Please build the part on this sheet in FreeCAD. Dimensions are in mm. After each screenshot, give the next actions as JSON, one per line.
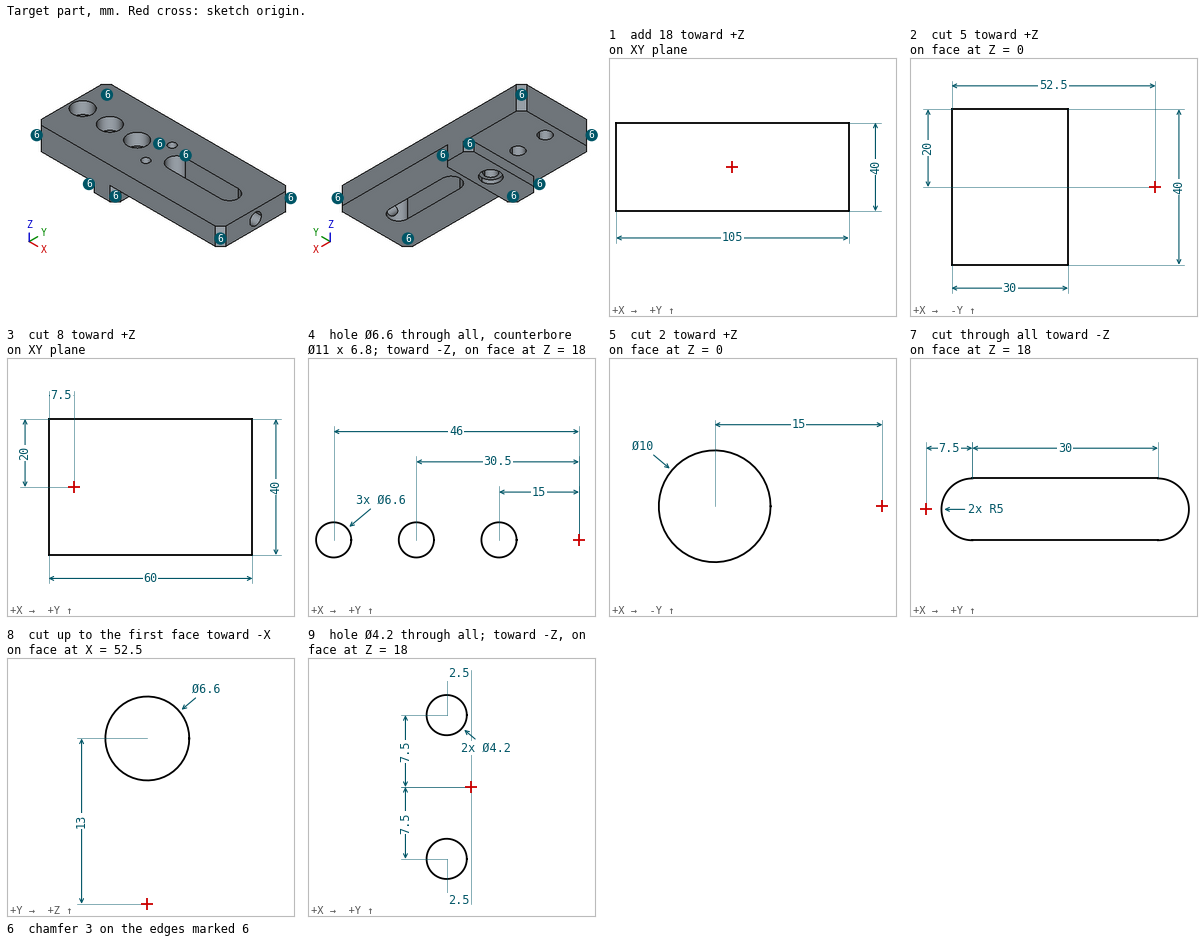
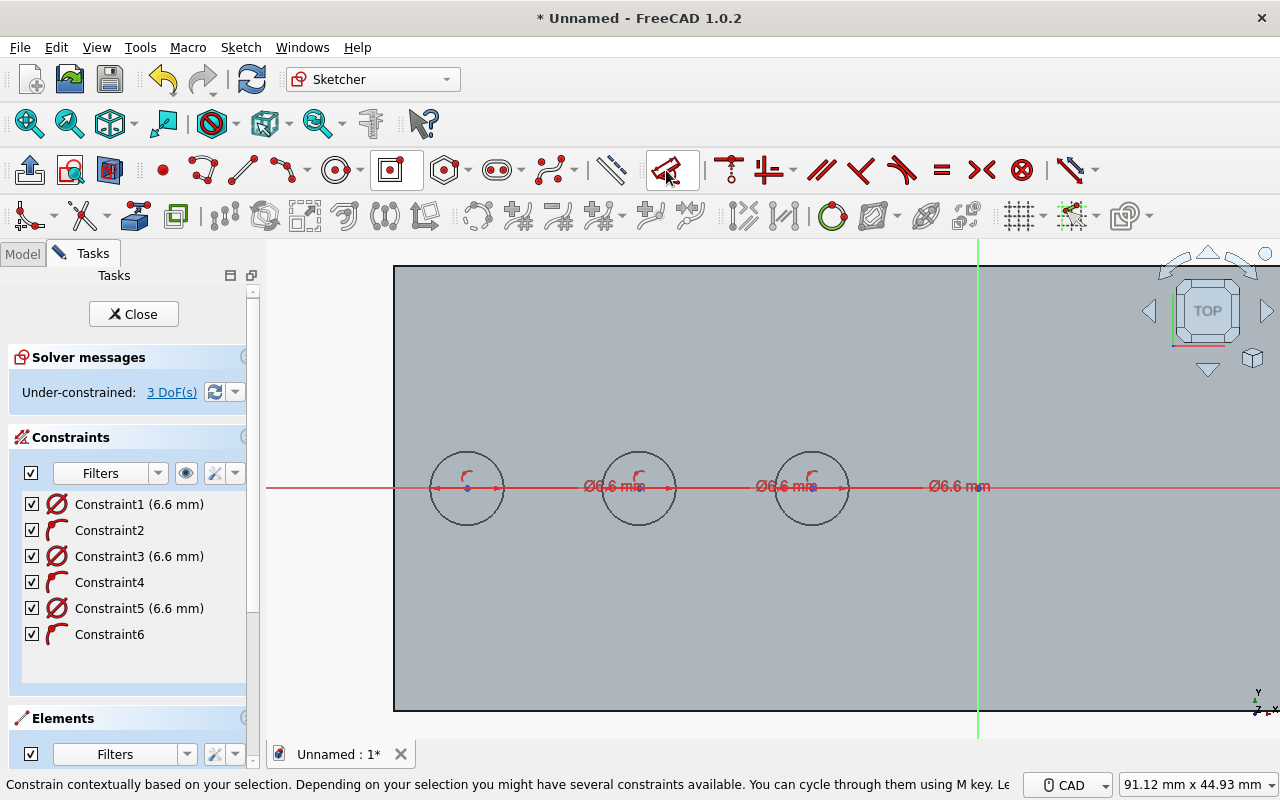
{"action": "left_click", "coordinate": [467, 488]}
{"action": "left_click", "coordinate": [723, 522]}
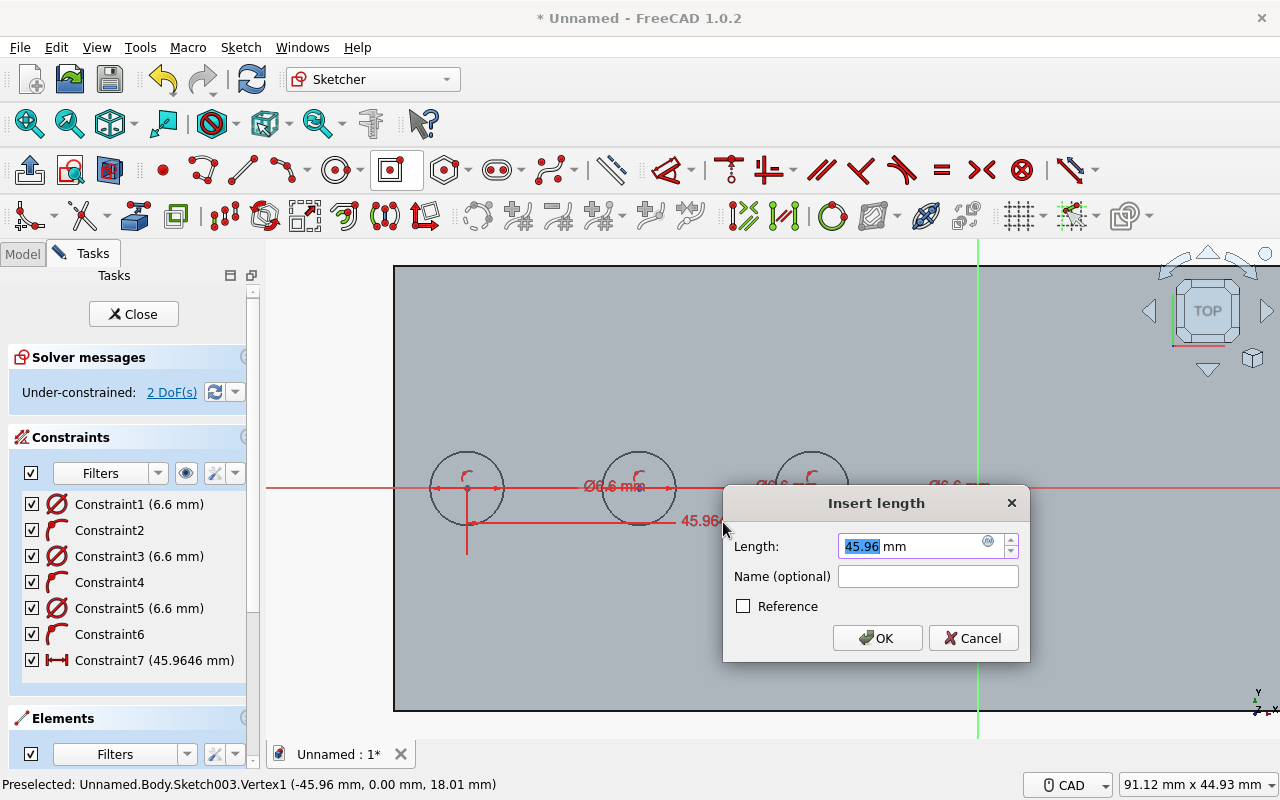
{"action": "type", "text": "46"}
{"action": "key", "text": "Return"}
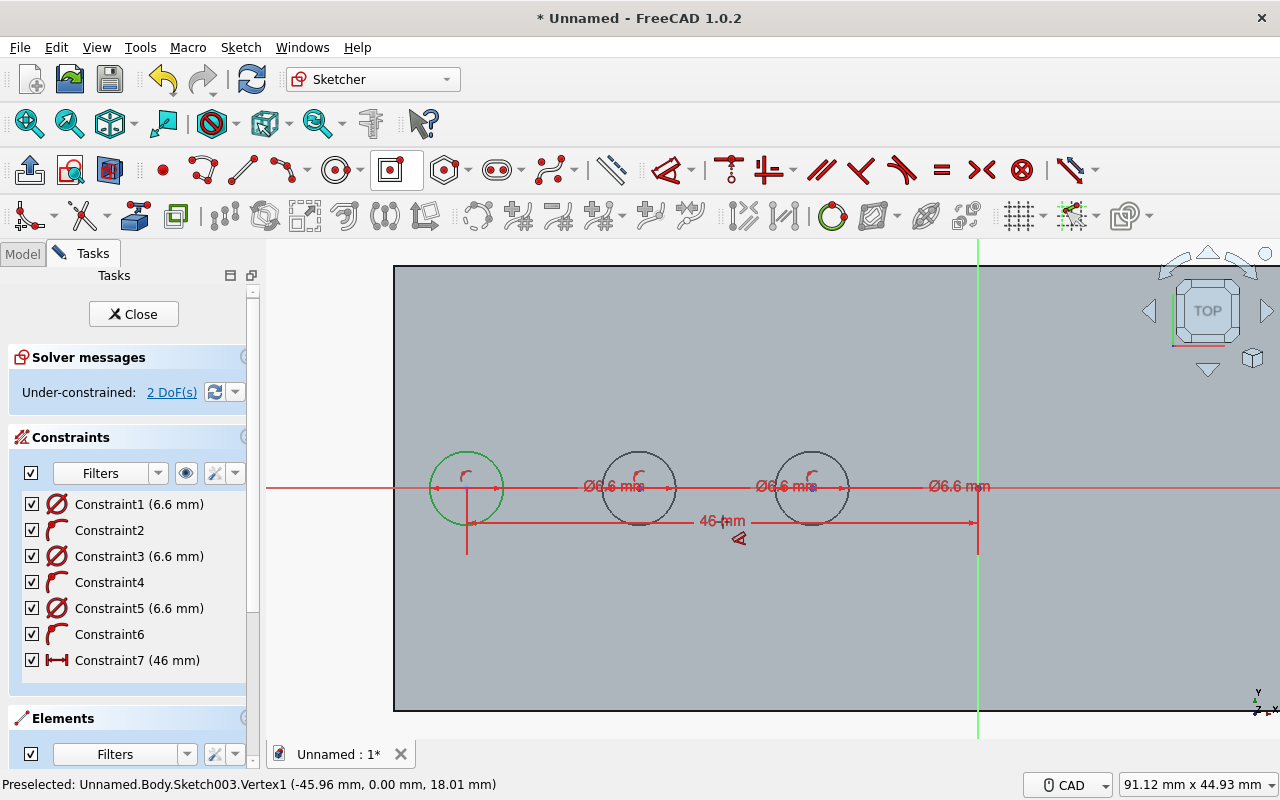
{"action": "left_click", "coordinate": [812, 488]}
{"action": "left_click", "coordinate": [895, 522]}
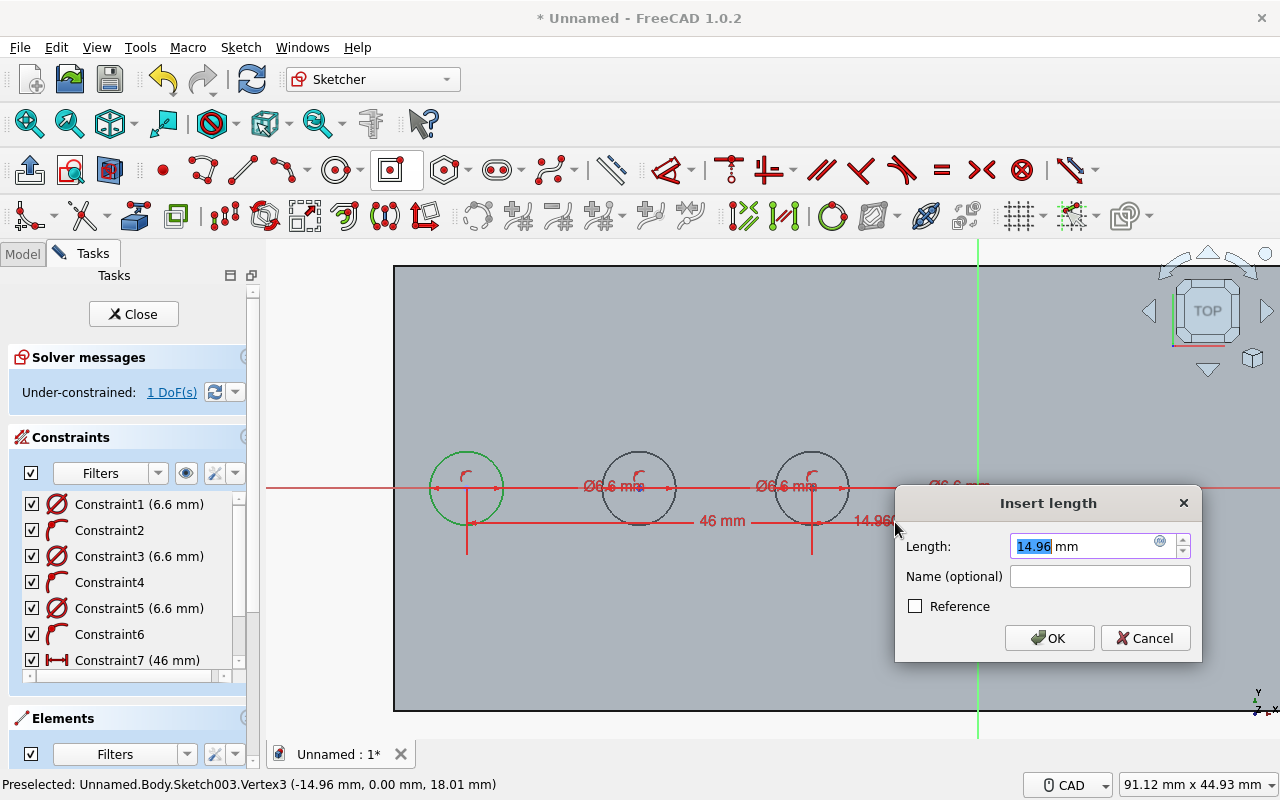
{"action": "type", "text": "15"}
{"action": "key", "text": "Return"}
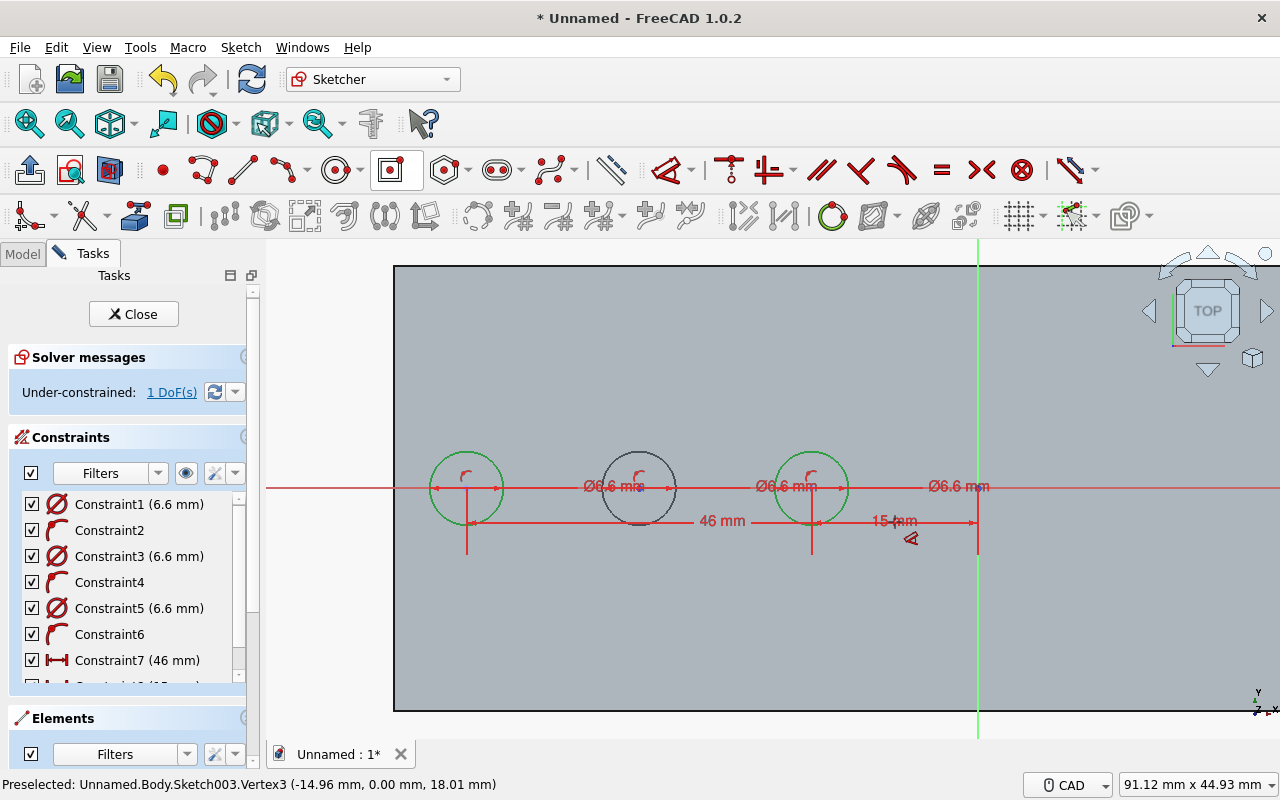
{"action": "left_click", "coordinate": [639, 488]}
{"action": "left_click", "coordinate": [731, 454]}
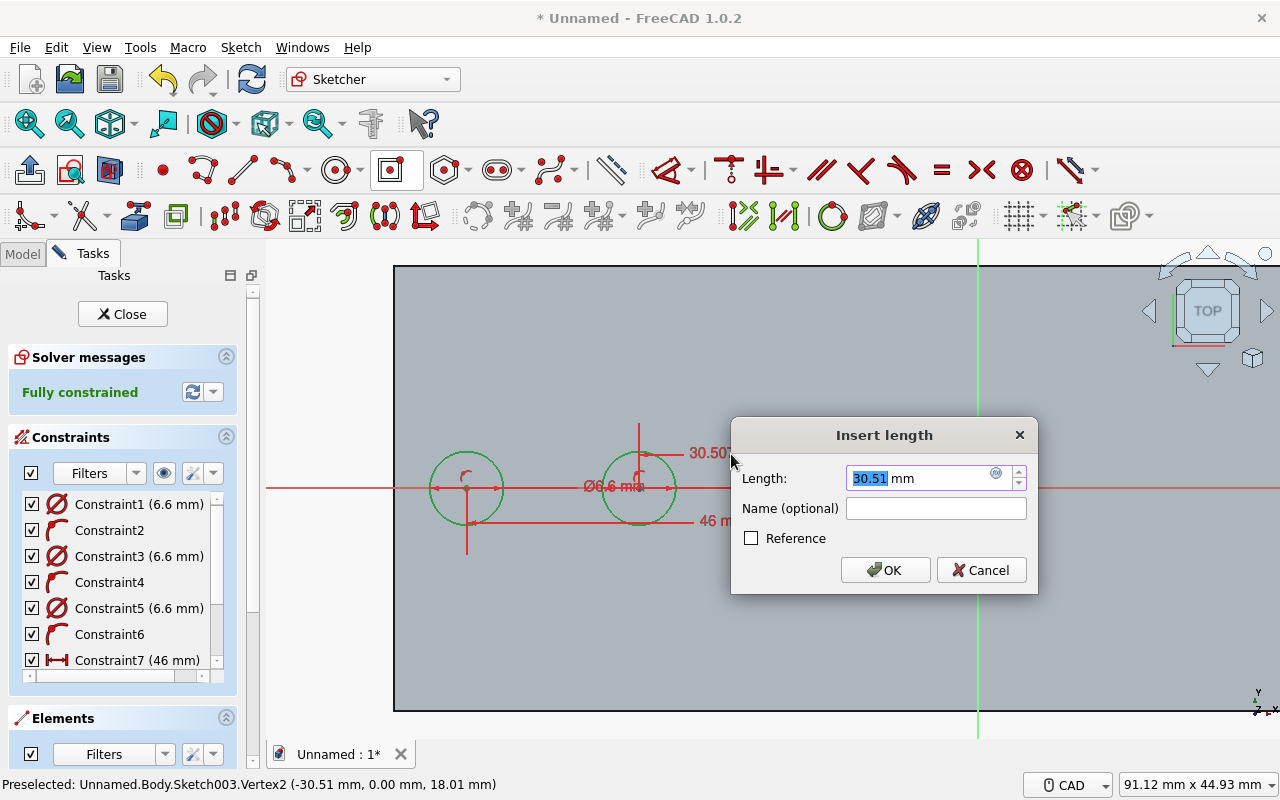
{"action": "type", "text": "30.5"}
{"action": "key", "text": "Return"}
{"action": "key", "text": "Escape"}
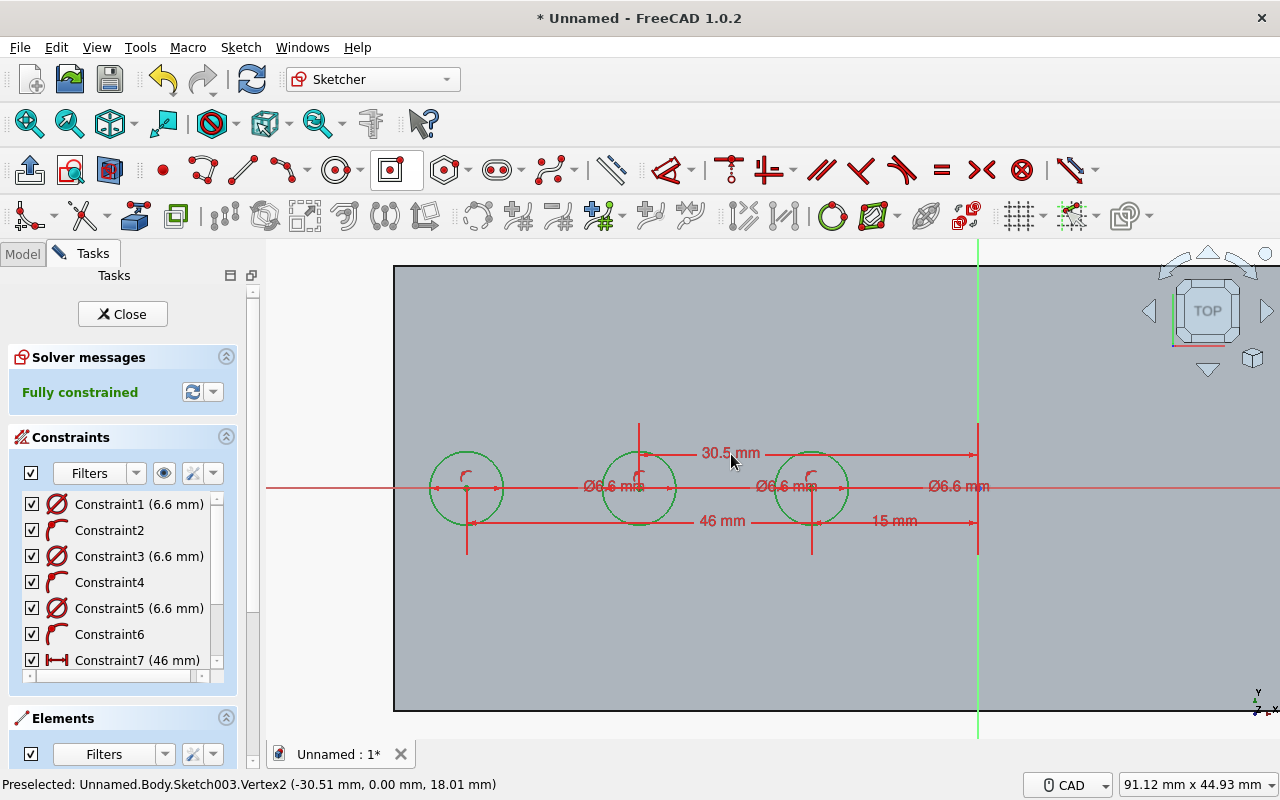
{"action": "left_click", "coordinate": [123, 314]}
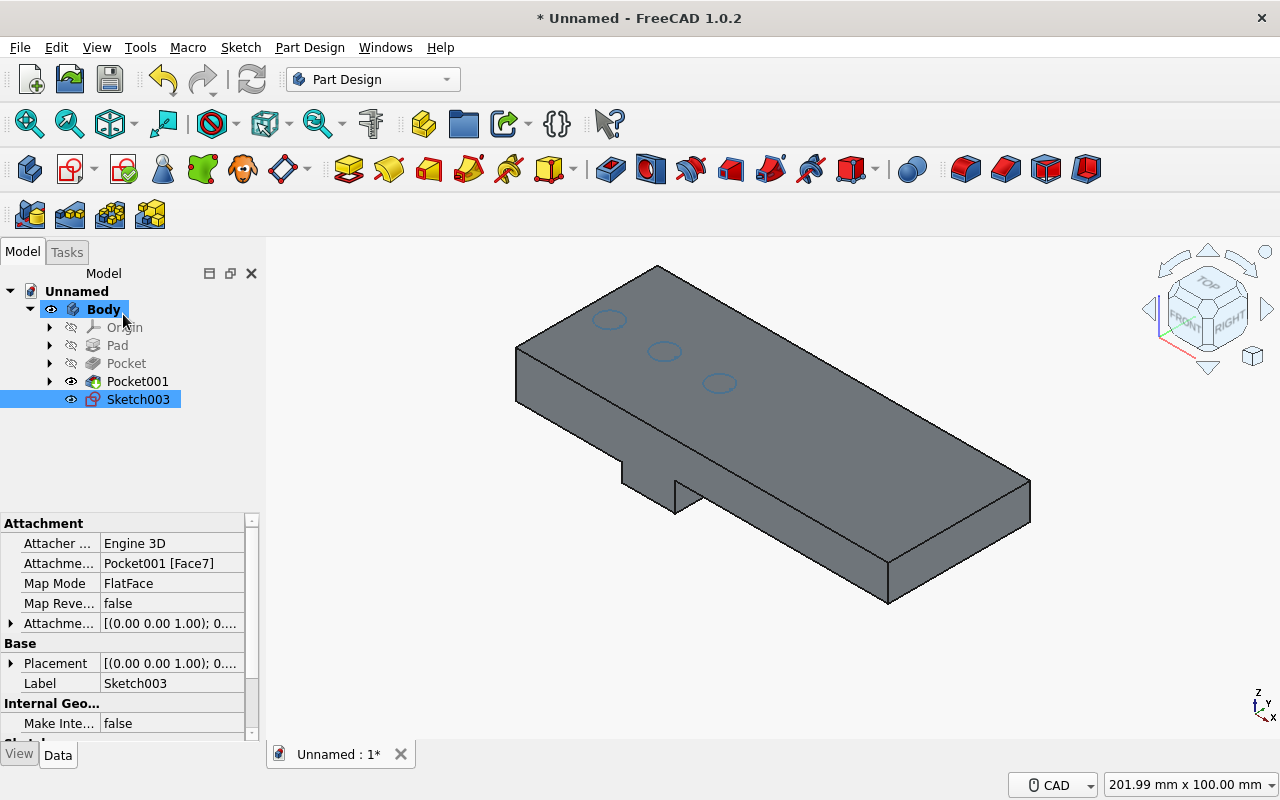
{"action": "left_click", "coordinate": [652, 170]}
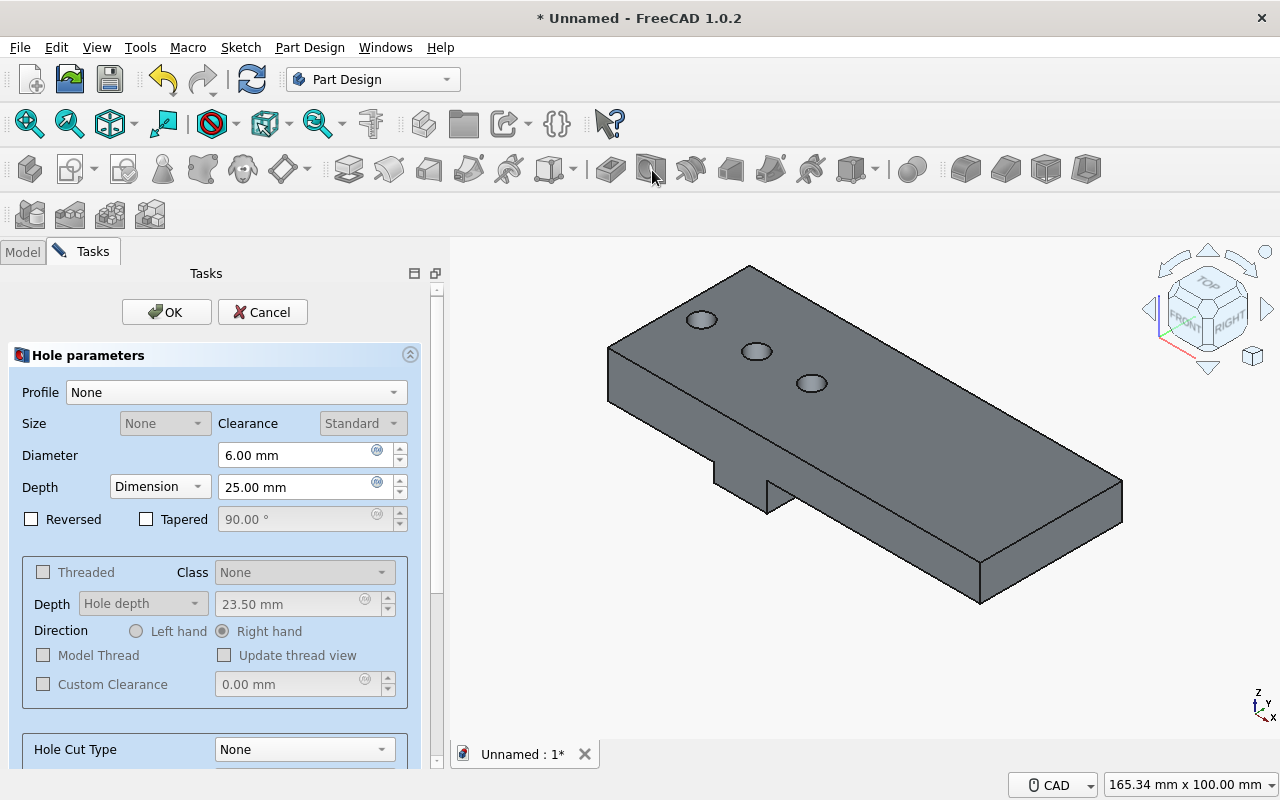
{"action": "triple_click", "coordinate": [305, 455]}